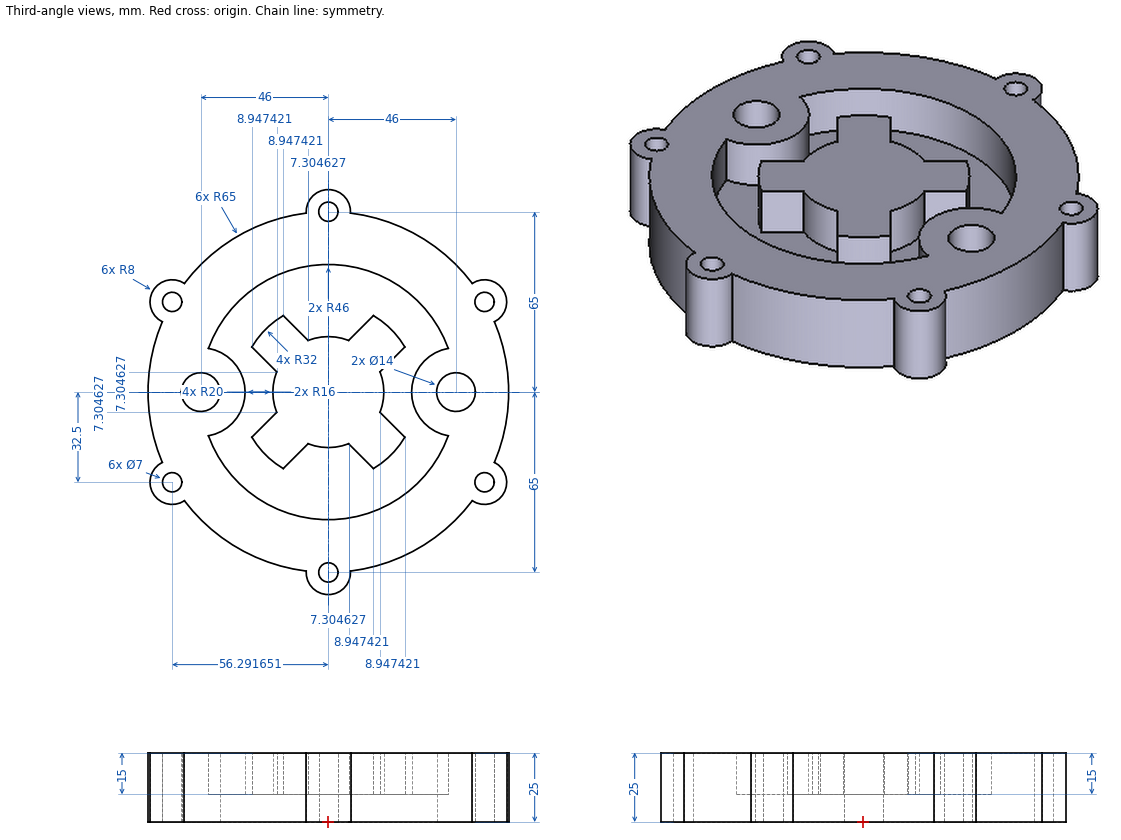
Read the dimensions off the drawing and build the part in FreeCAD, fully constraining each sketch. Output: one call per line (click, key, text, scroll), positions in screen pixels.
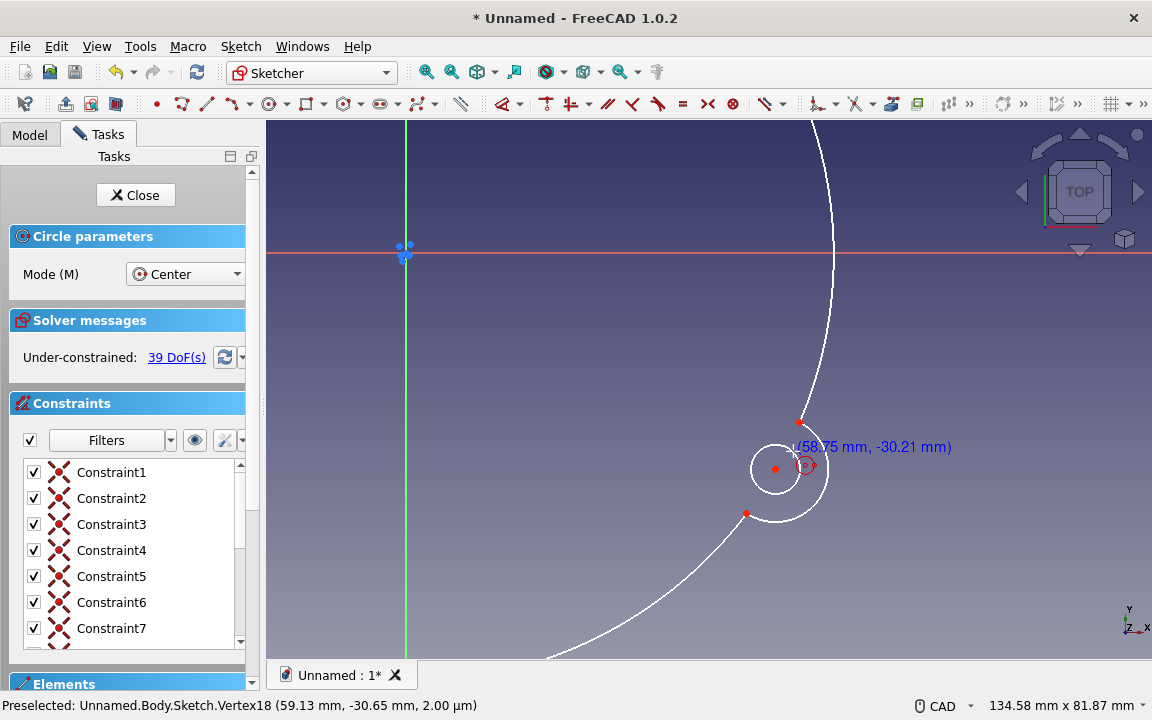
scroll(777, 469, down, 5)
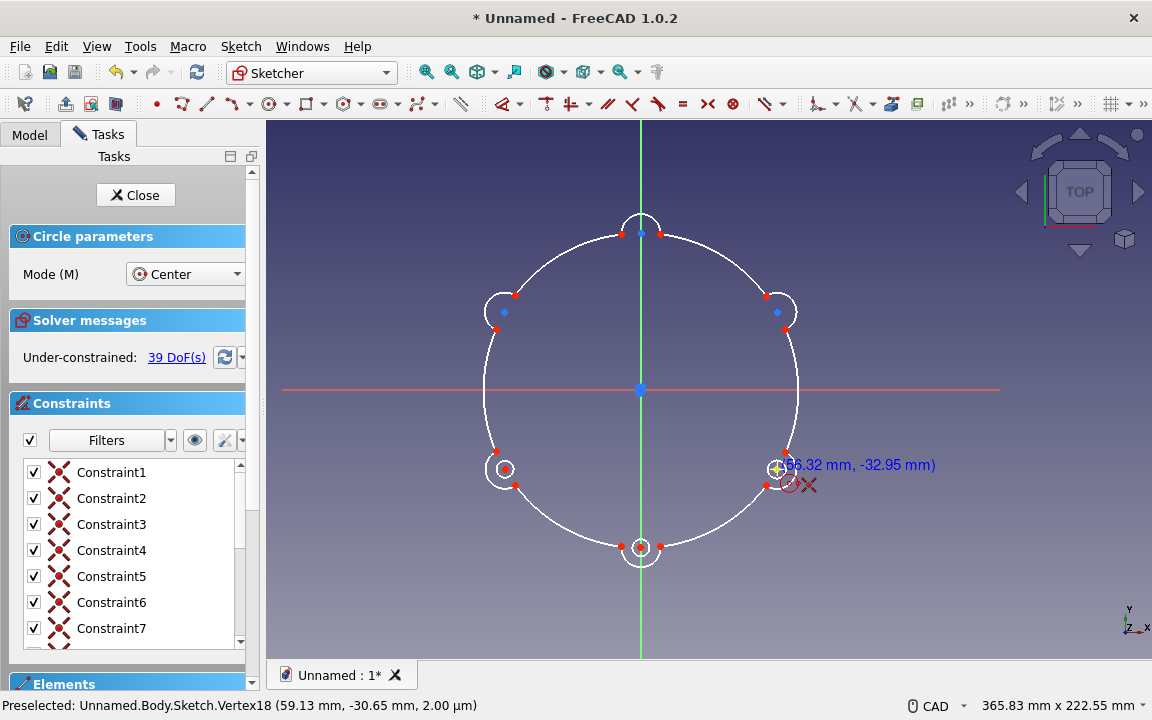
scroll(505, 311, up, 5)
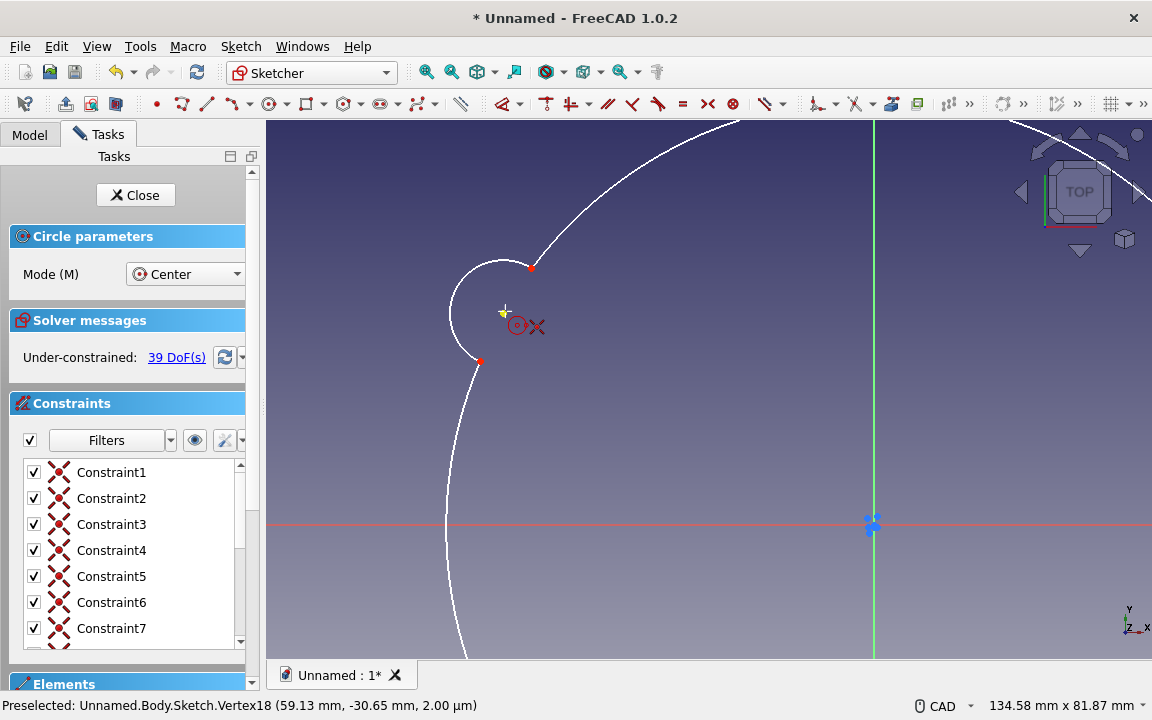
click(504, 311)
click(520, 295)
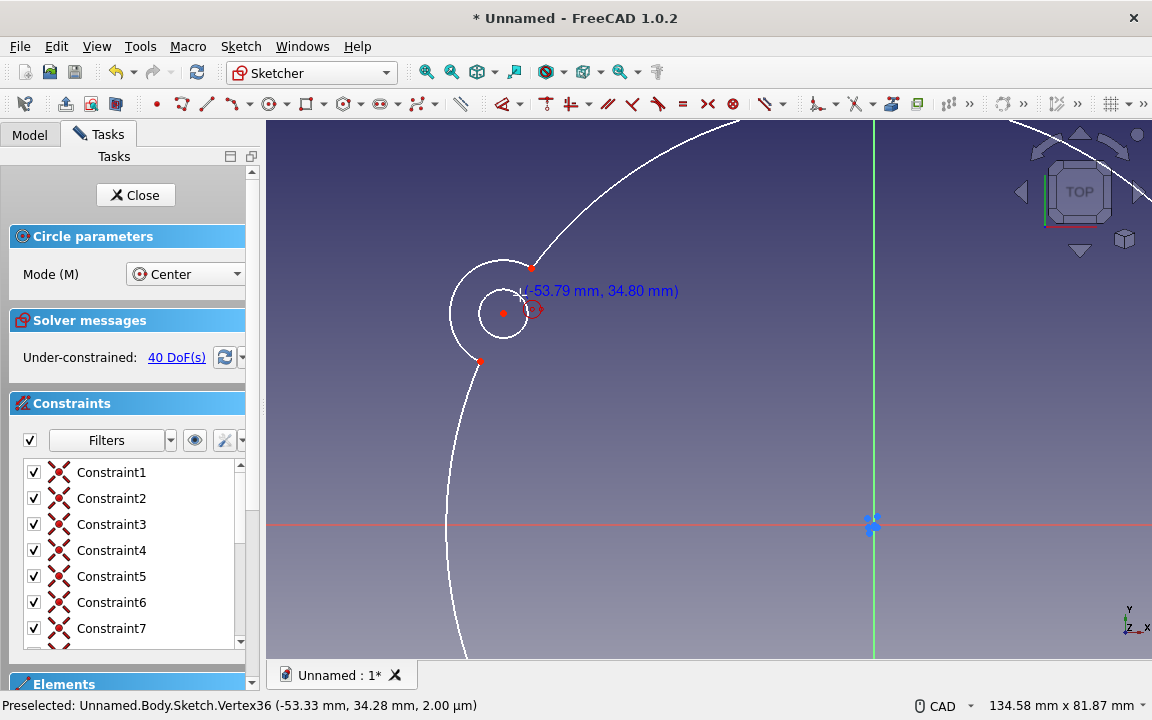
scroll(505, 311, down, 5)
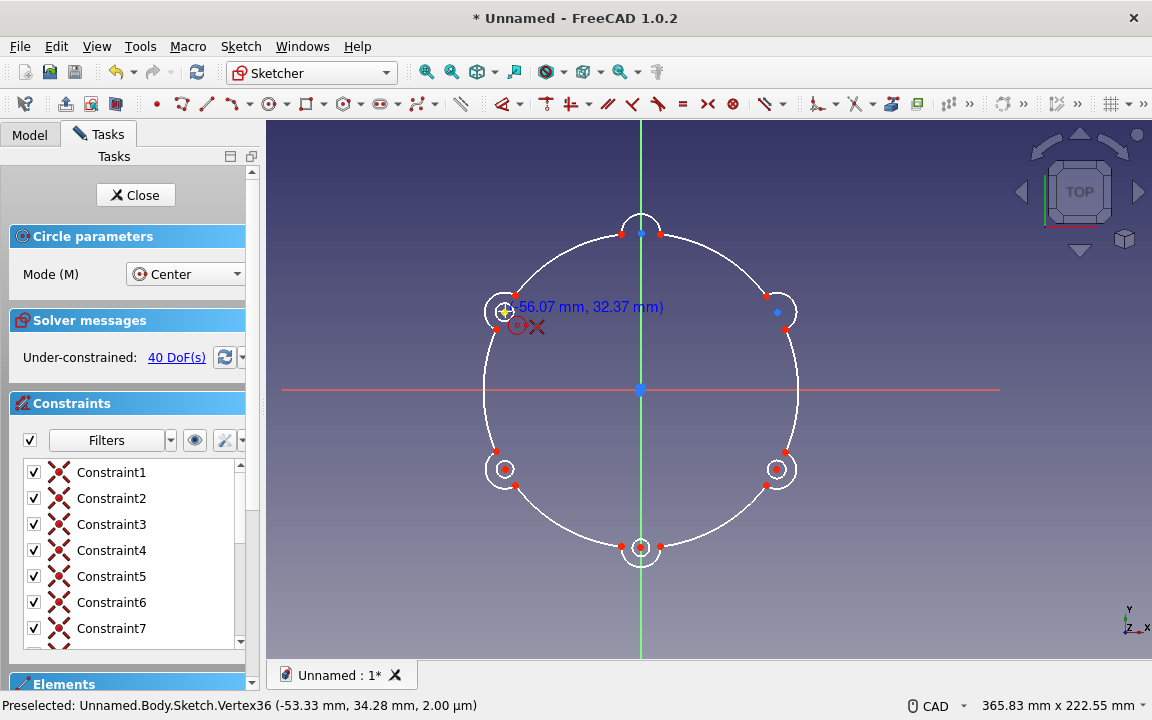
scroll(777, 311, up, 5)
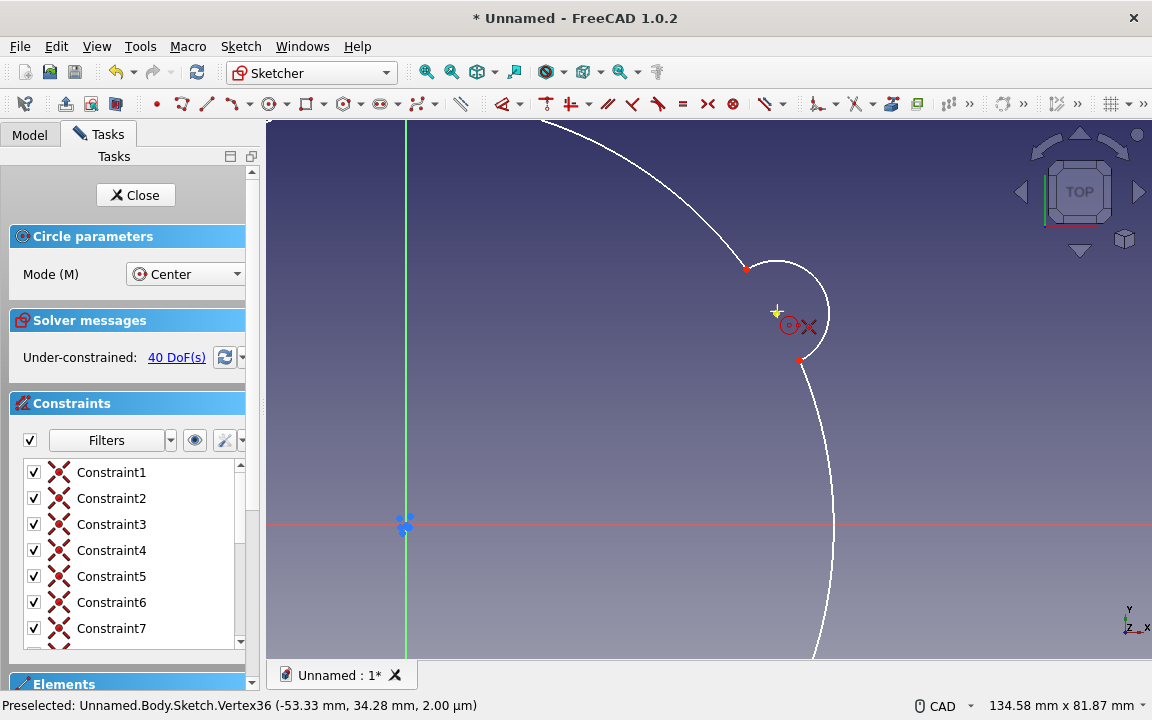
click(777, 311)
click(793, 295)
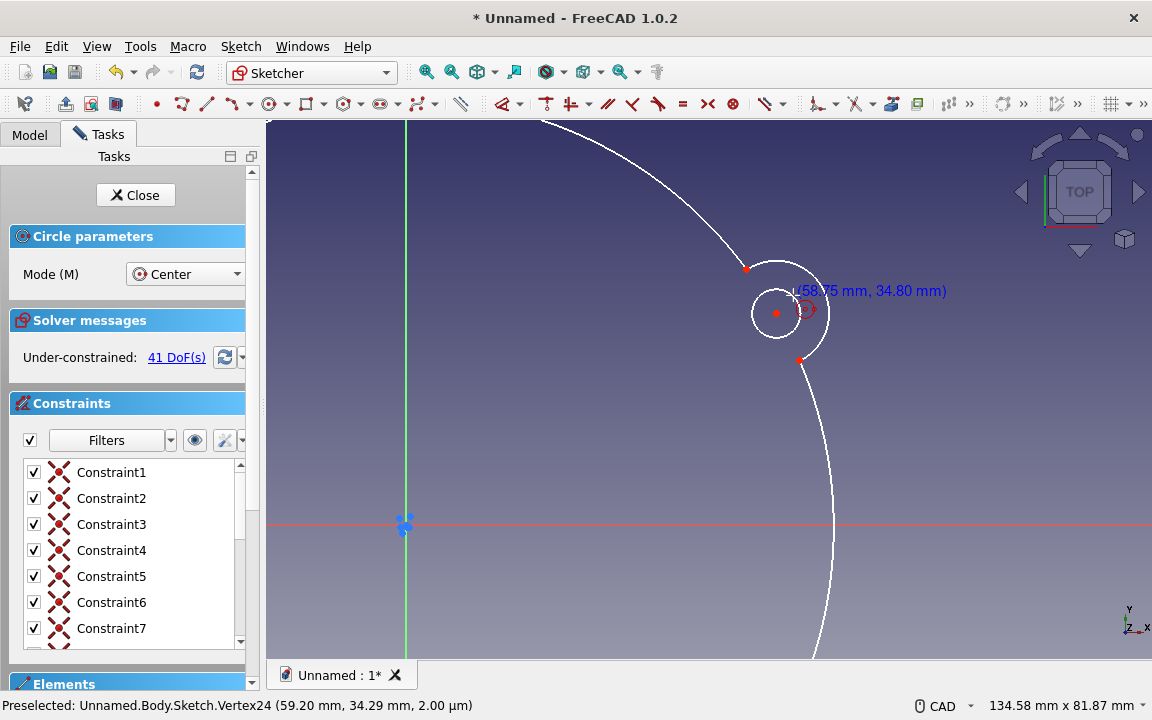
scroll(777, 311, down, 5)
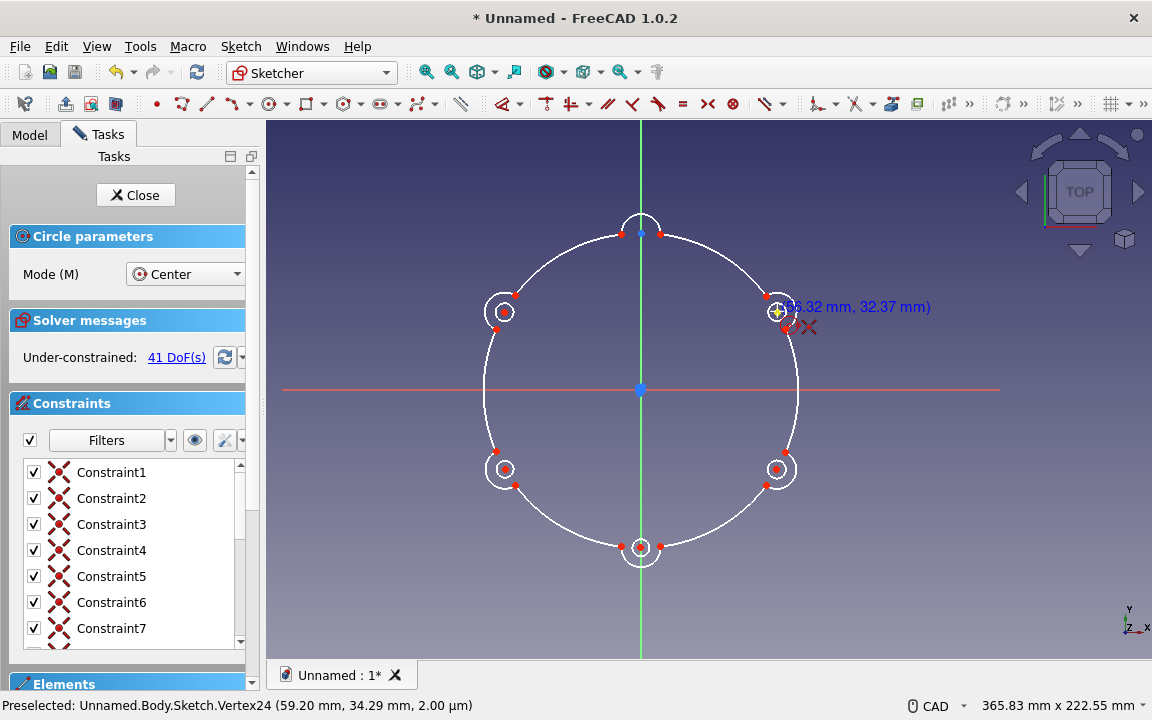
scroll(641, 233, up, 5)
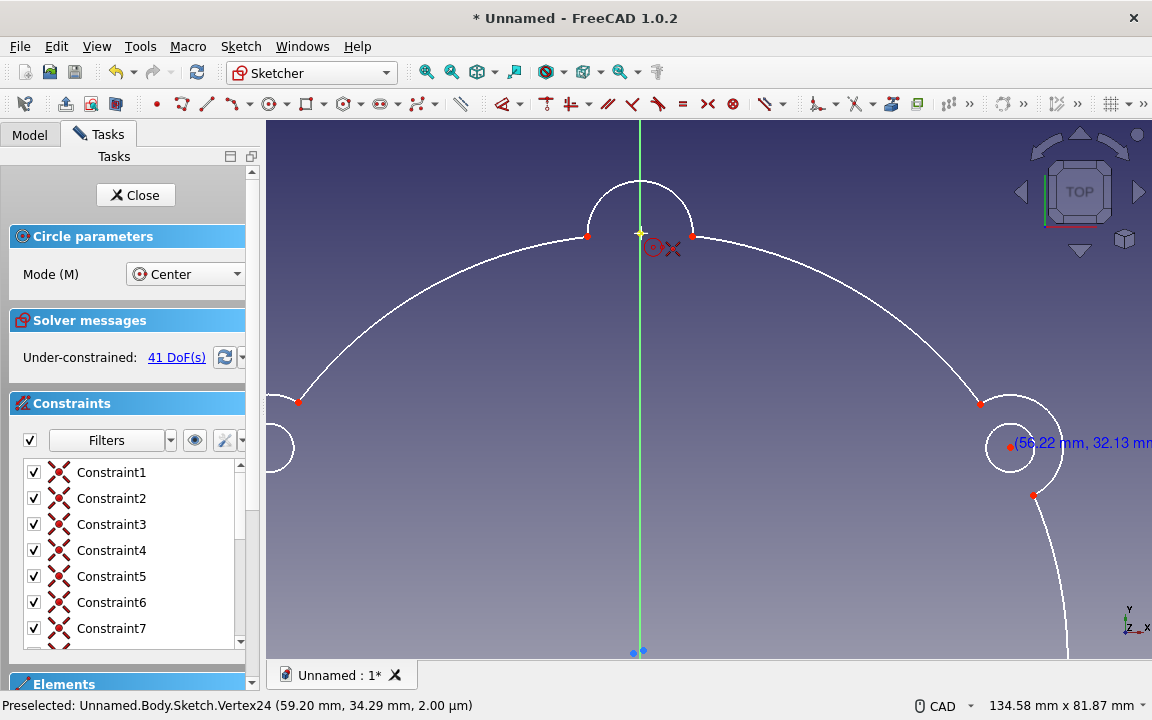
click(640, 231)
click(656, 215)
key(Escape)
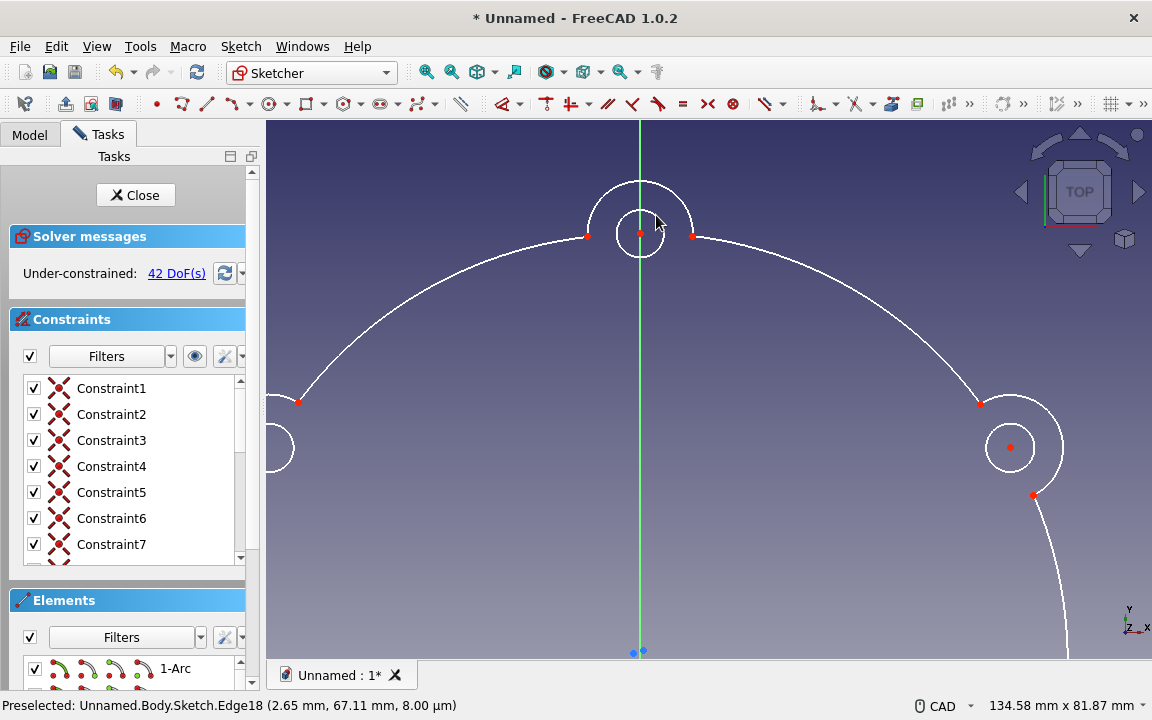
scroll(641, 232, down, 5)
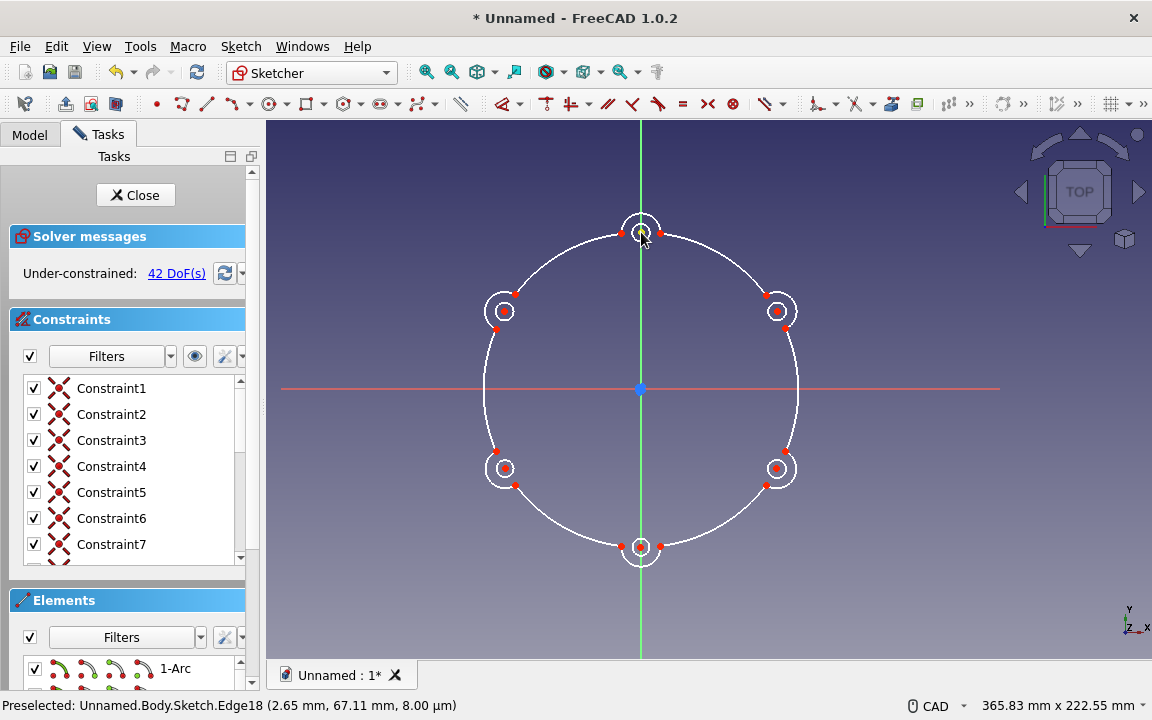
click(486, 365)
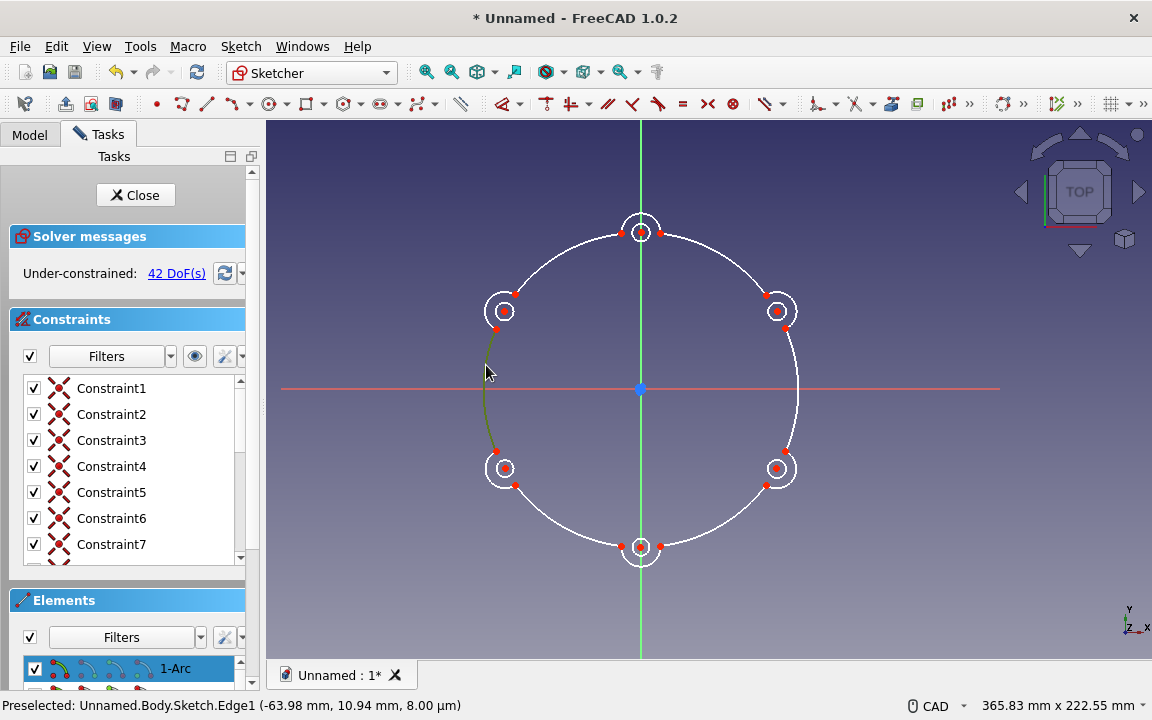
click(542, 512)